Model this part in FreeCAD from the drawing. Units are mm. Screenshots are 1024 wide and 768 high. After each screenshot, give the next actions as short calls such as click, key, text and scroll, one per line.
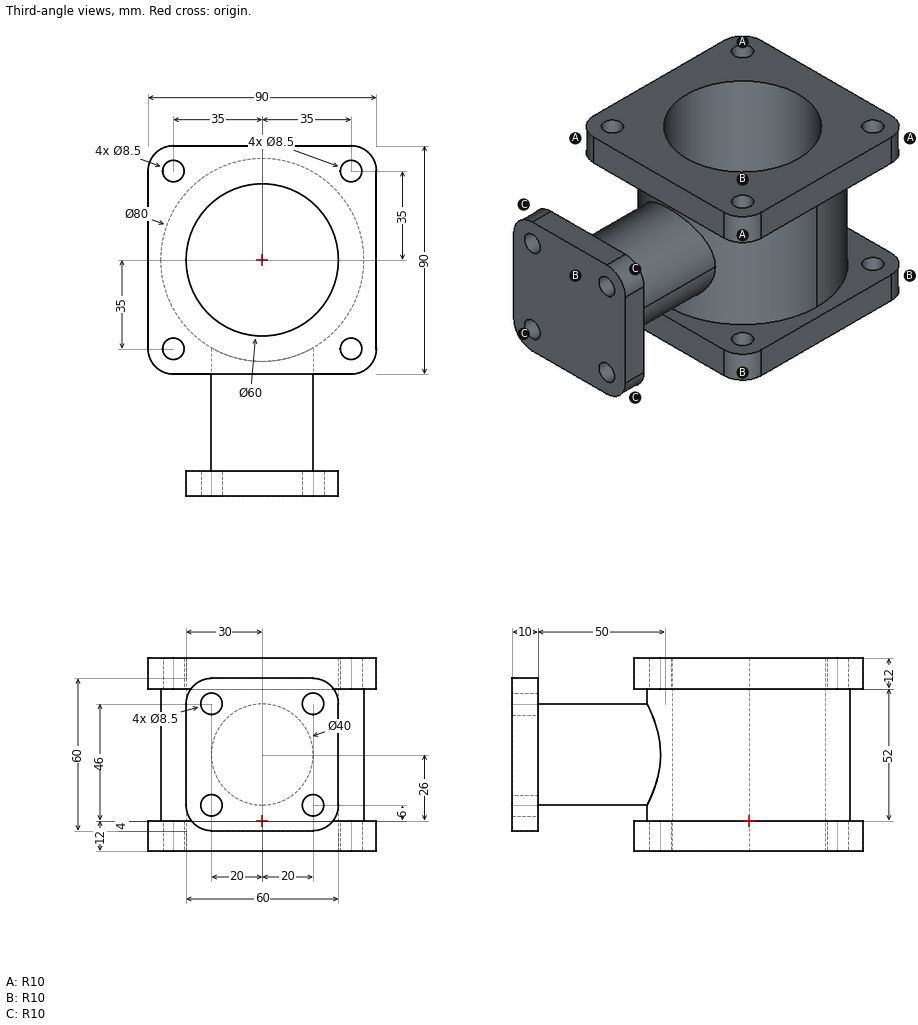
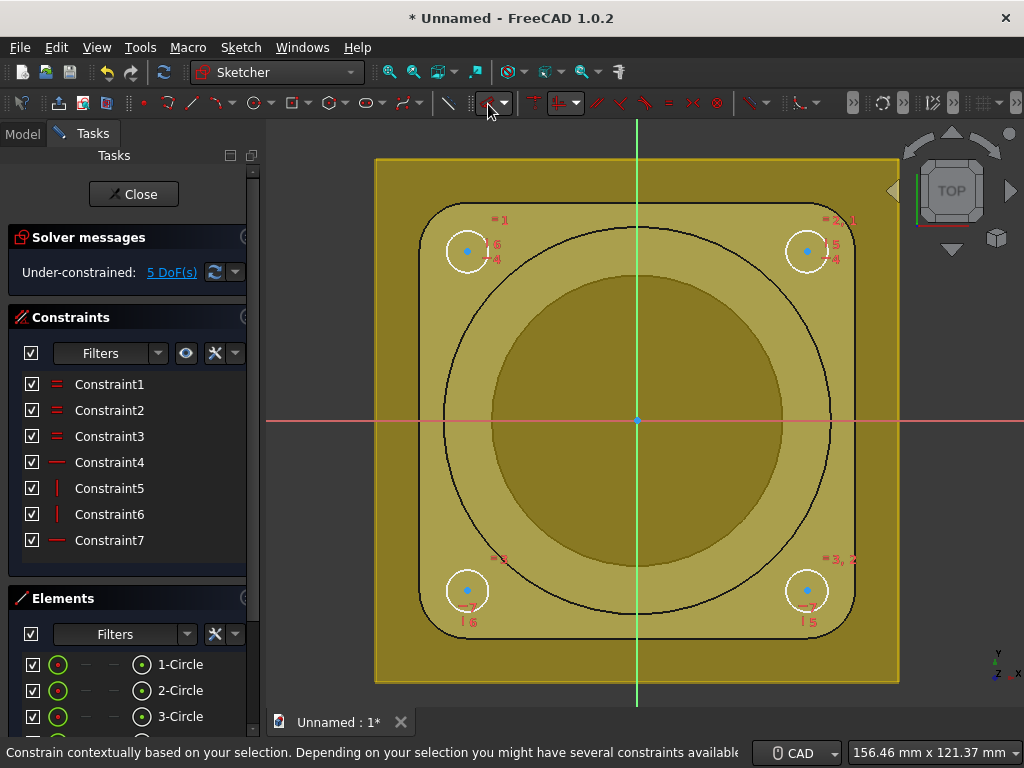
click(482, 237)
click(504, 214)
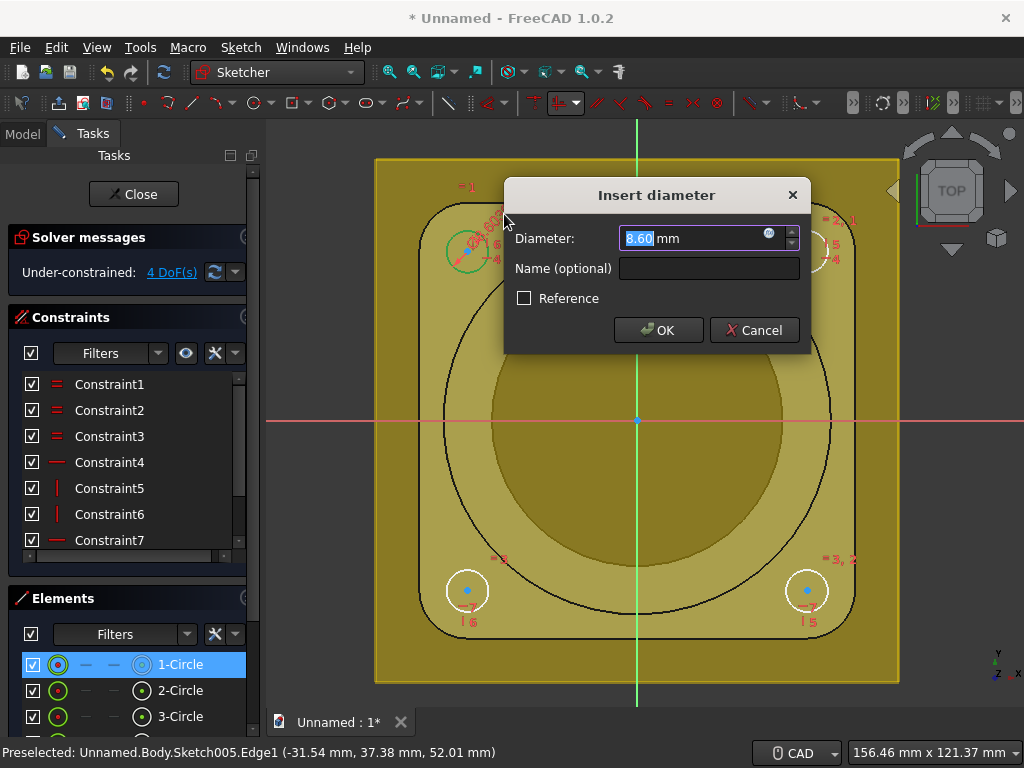
text(8.5)
key(Return)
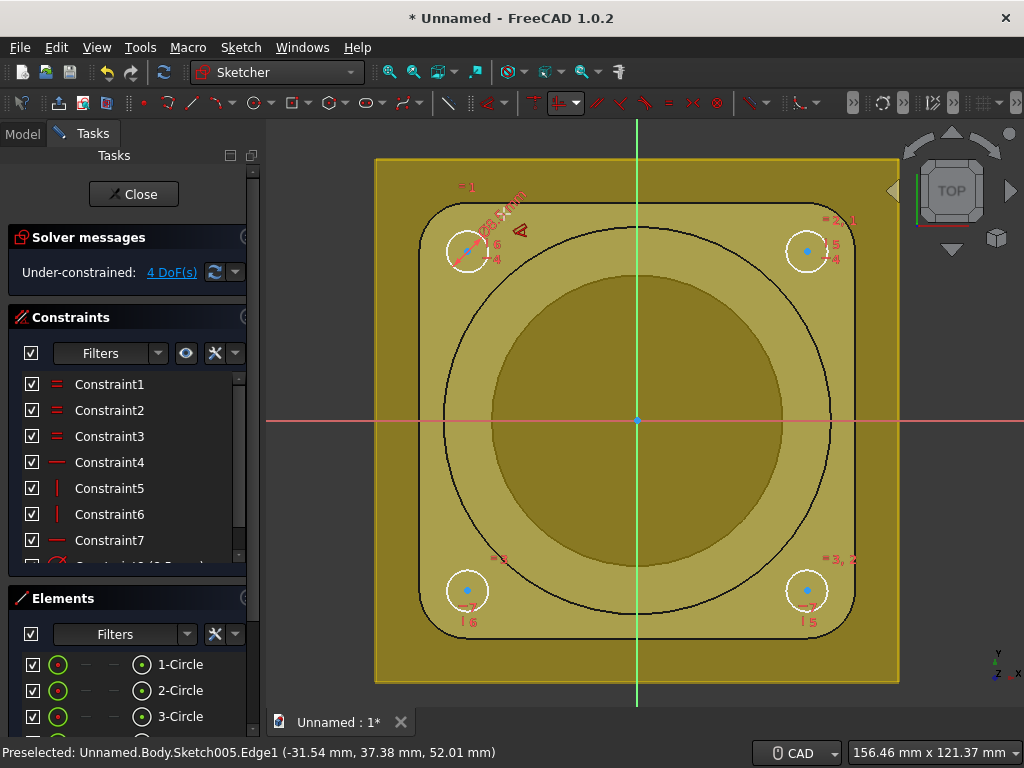
click(468, 252)
click(591, 218)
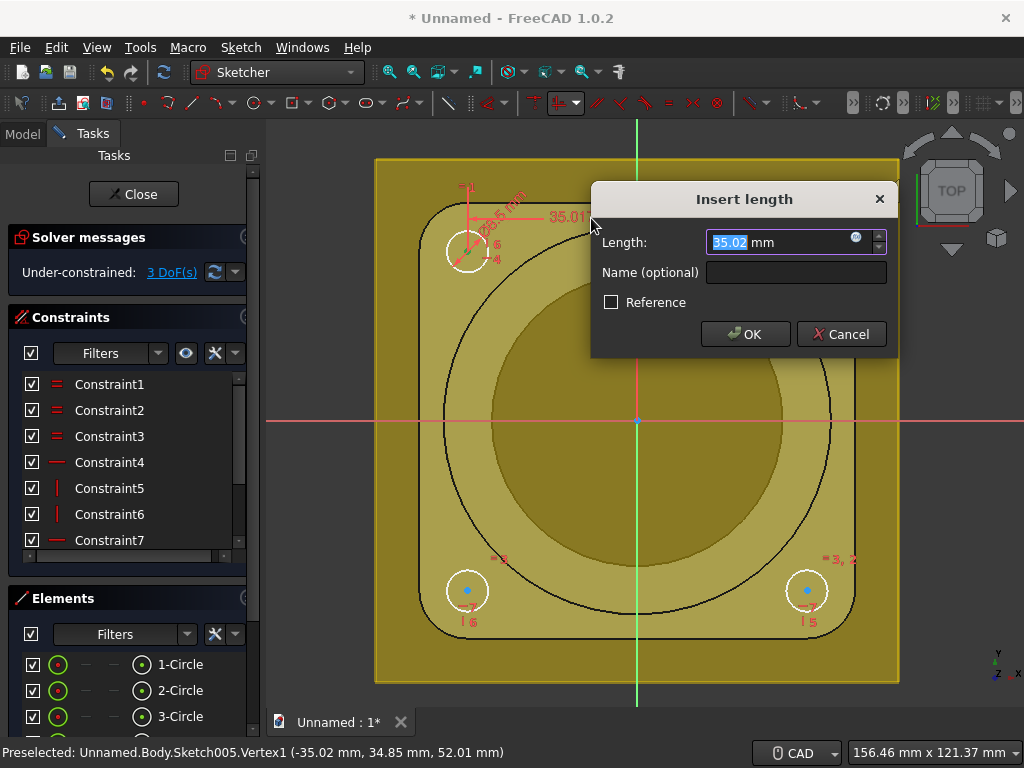
text(35)
key(Return)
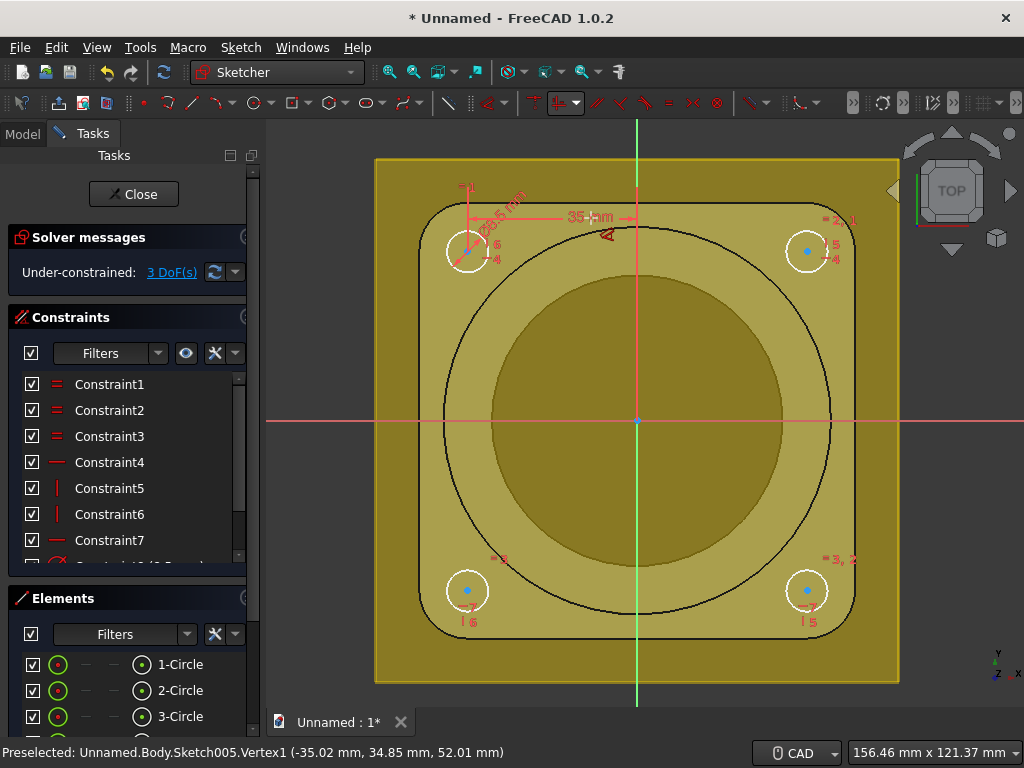
click(468, 252)
click(434, 336)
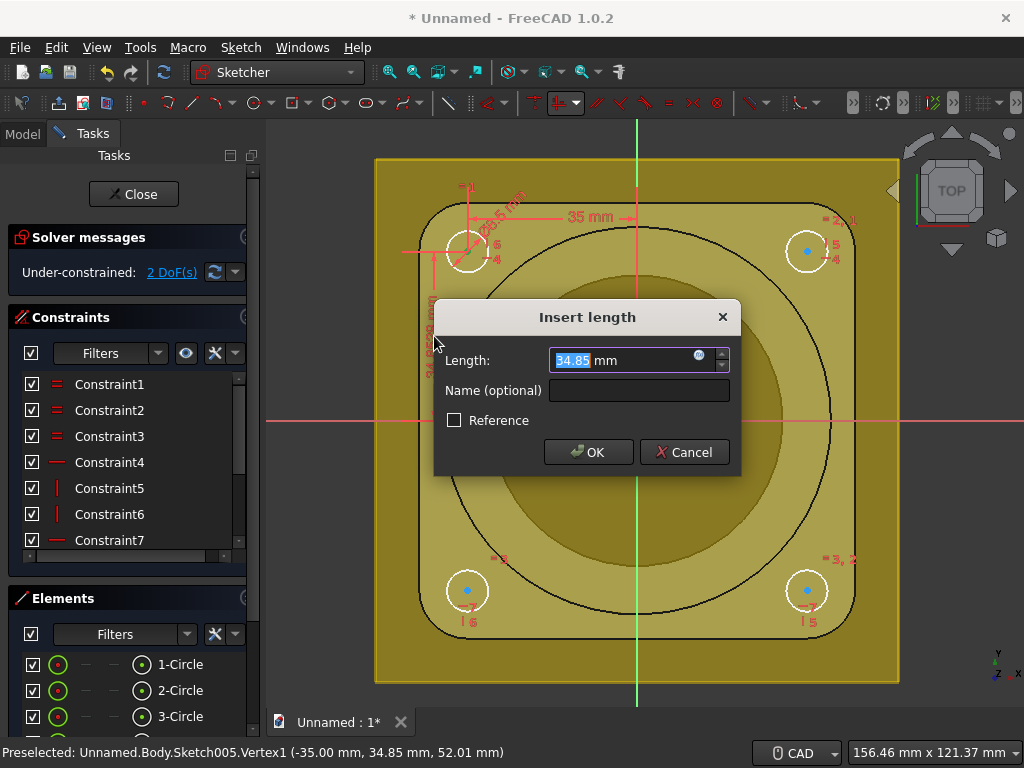
text(35)
key(Return)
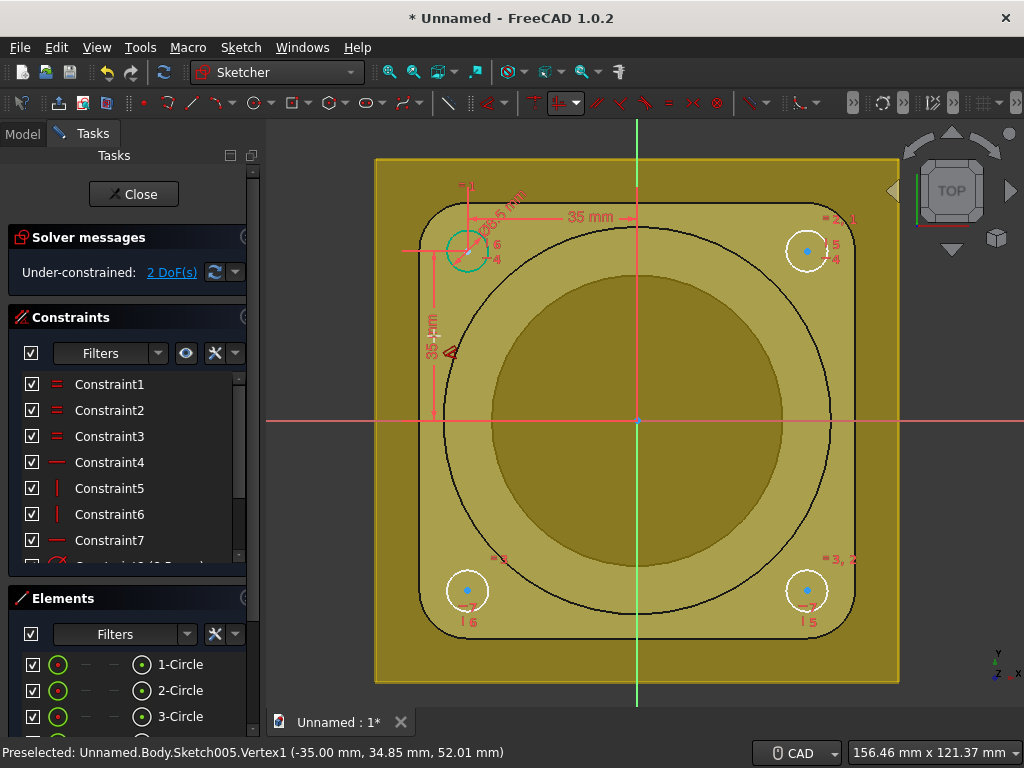
click(807, 251)
click(722, 217)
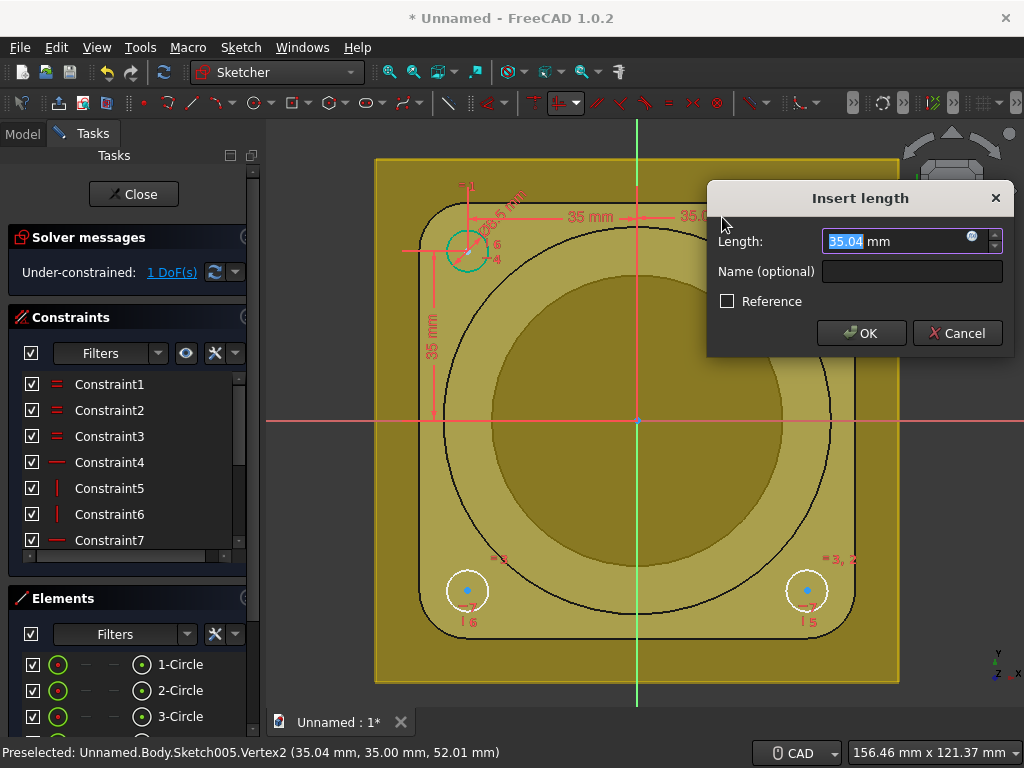
text(35)
key(Return)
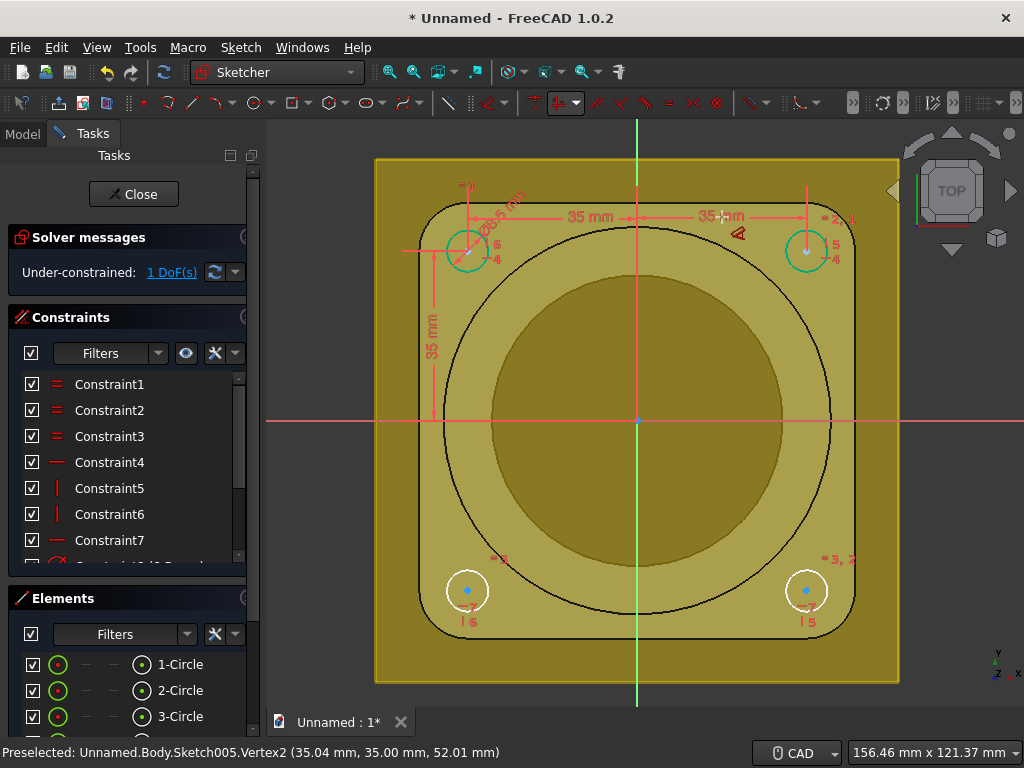
click(807, 591)
click(841, 506)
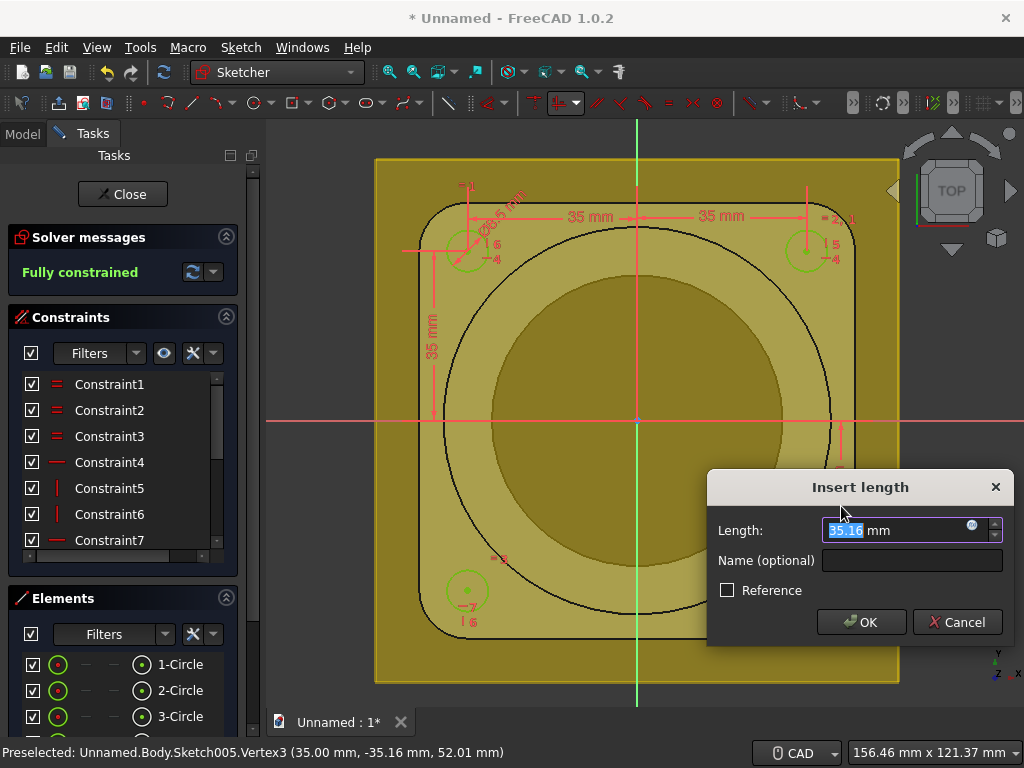
text(35)
key(Return)
key(Escape)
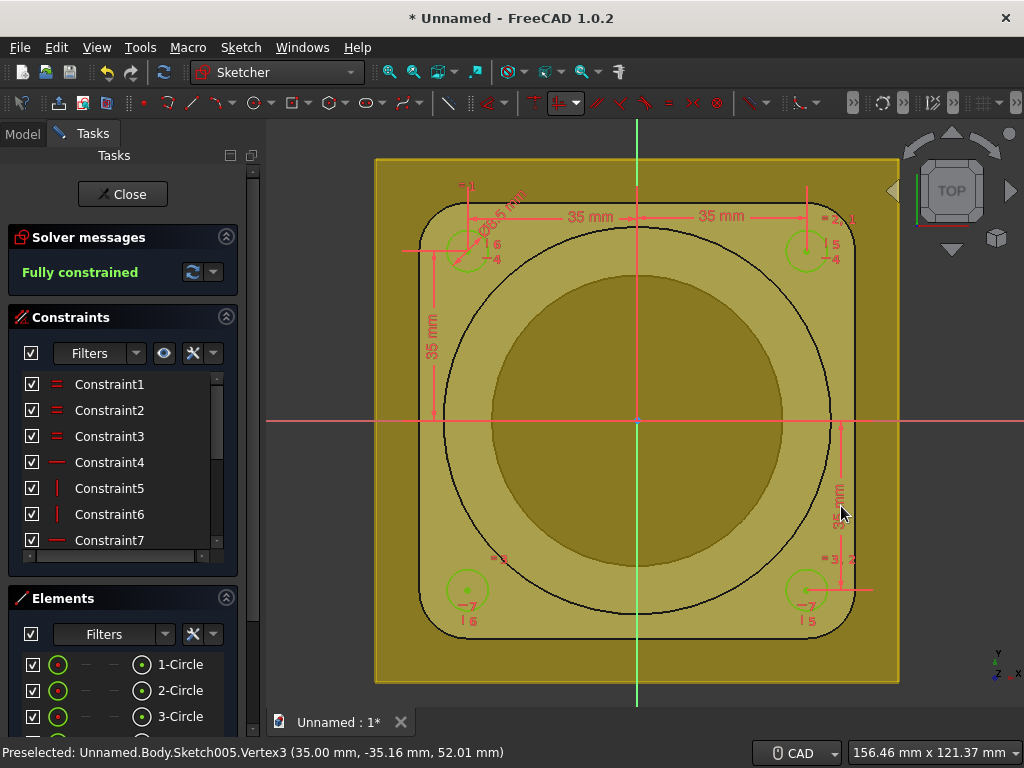
click(123, 194)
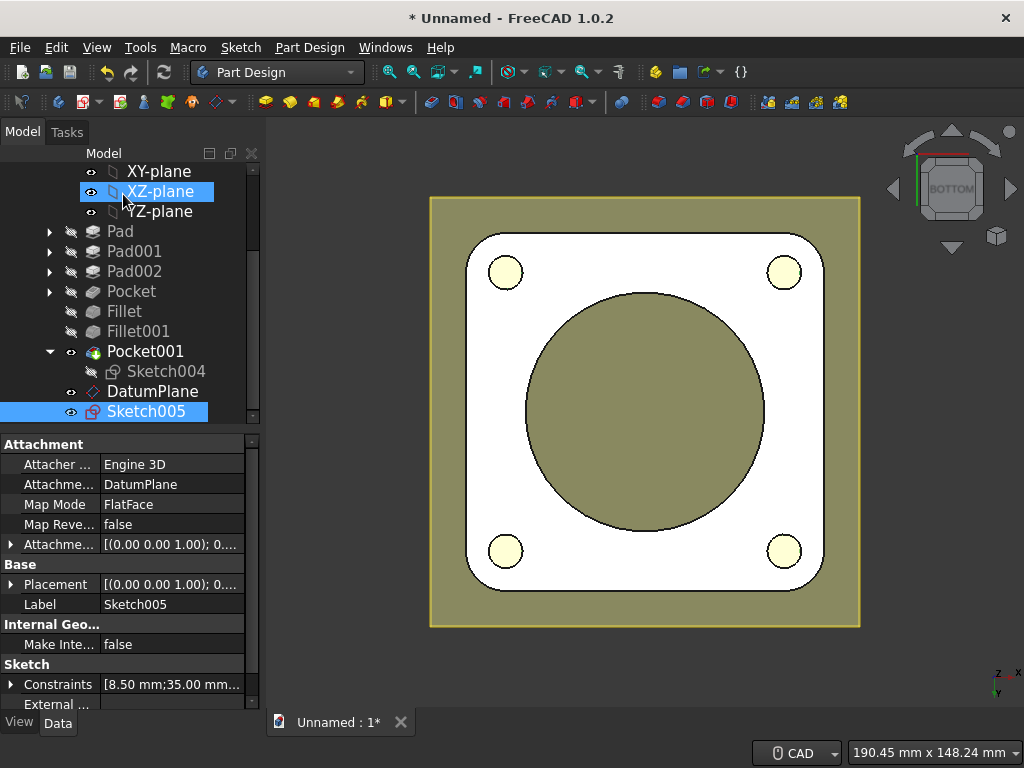
click(432, 102)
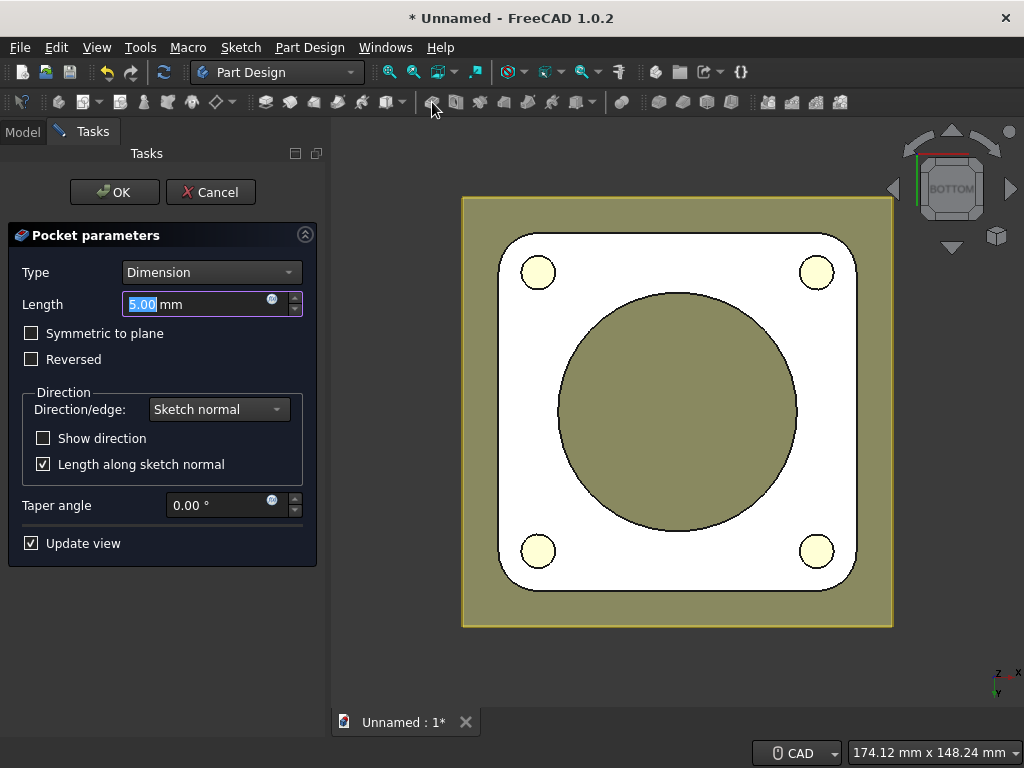
text(12)
key(Tab)